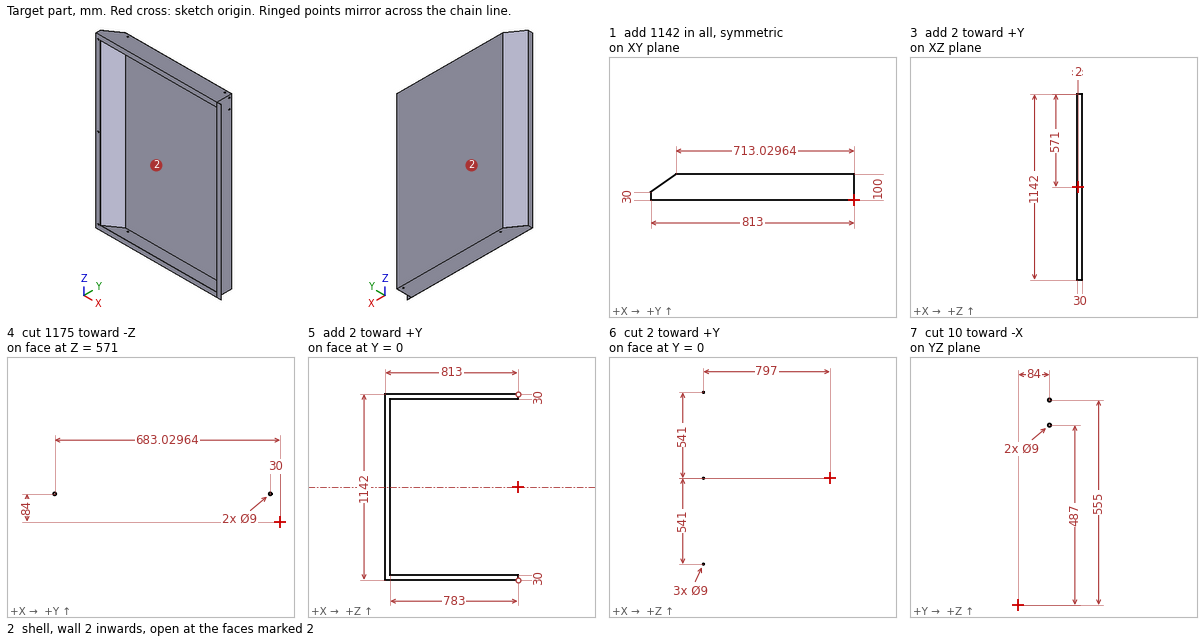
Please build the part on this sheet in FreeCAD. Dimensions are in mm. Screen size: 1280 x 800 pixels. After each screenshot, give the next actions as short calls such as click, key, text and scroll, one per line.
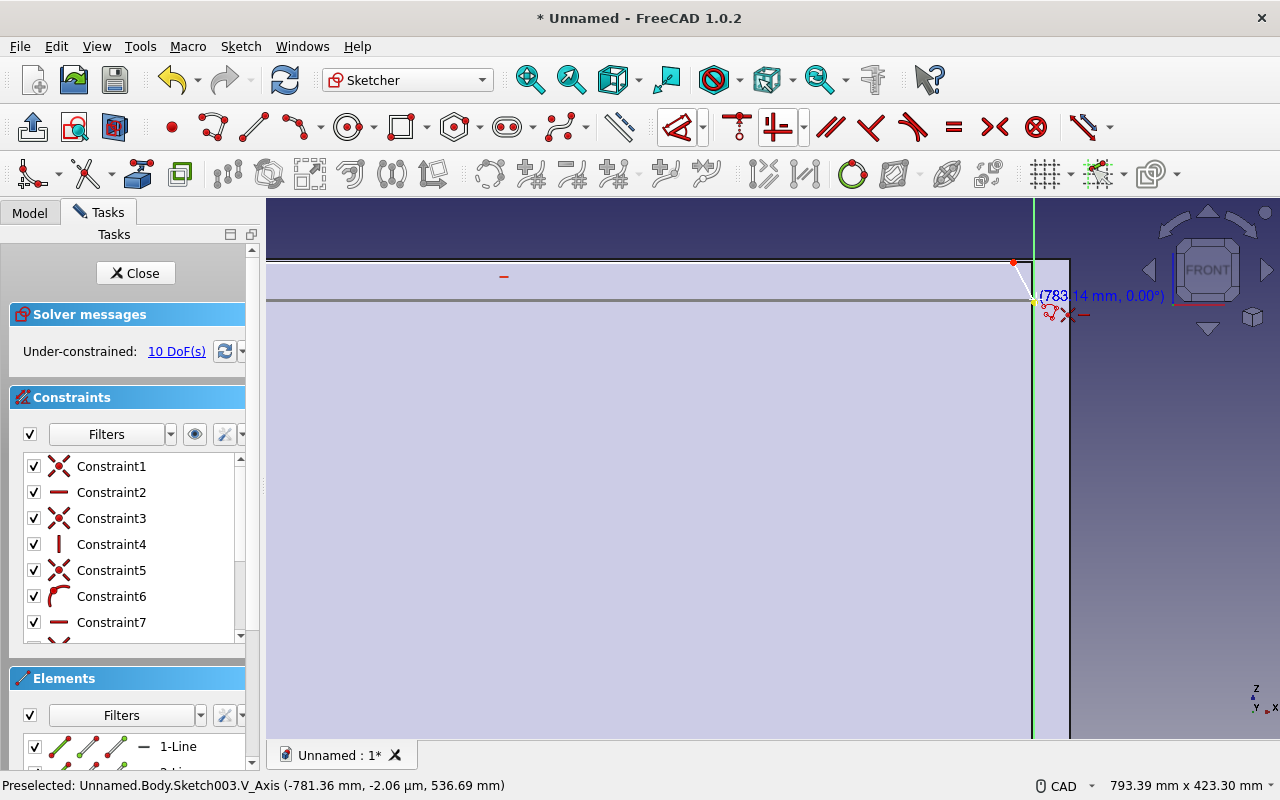
click(1035, 302)
key(Escape)
key(Escape)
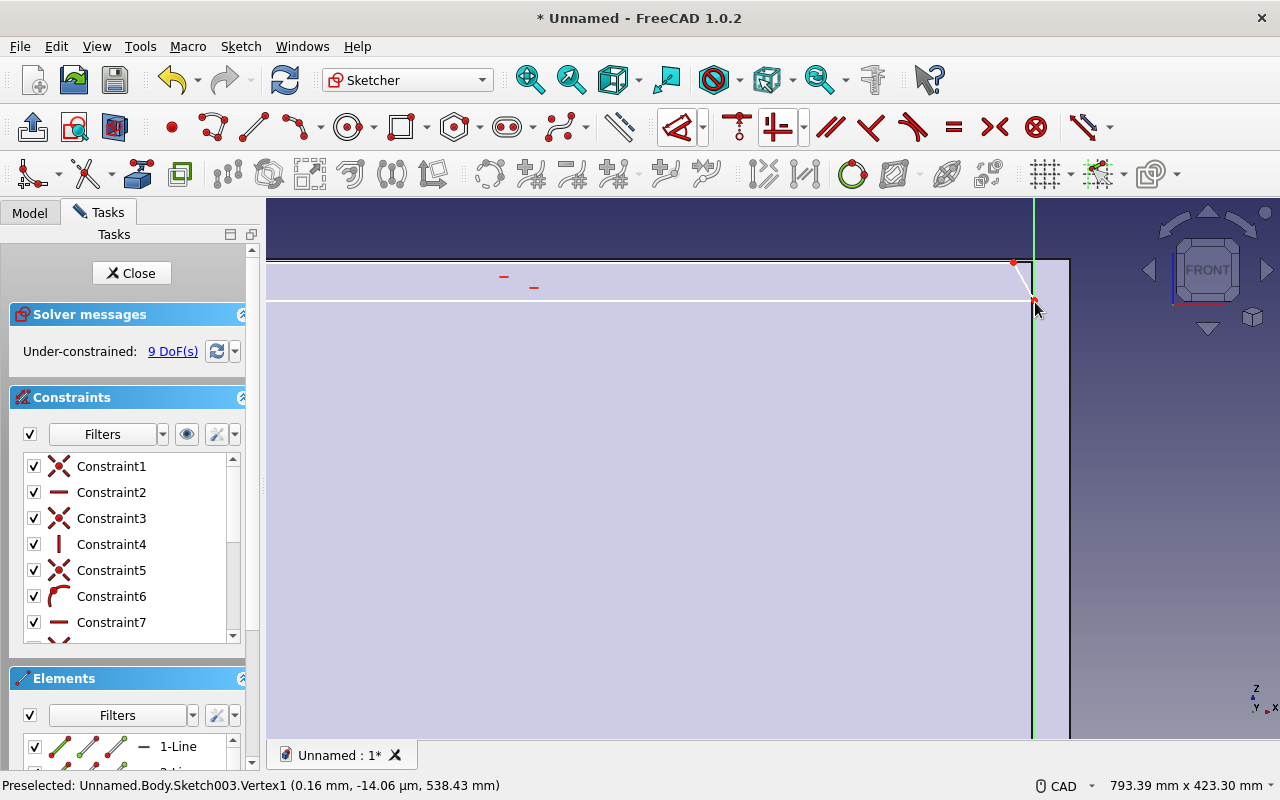
click(1020, 274)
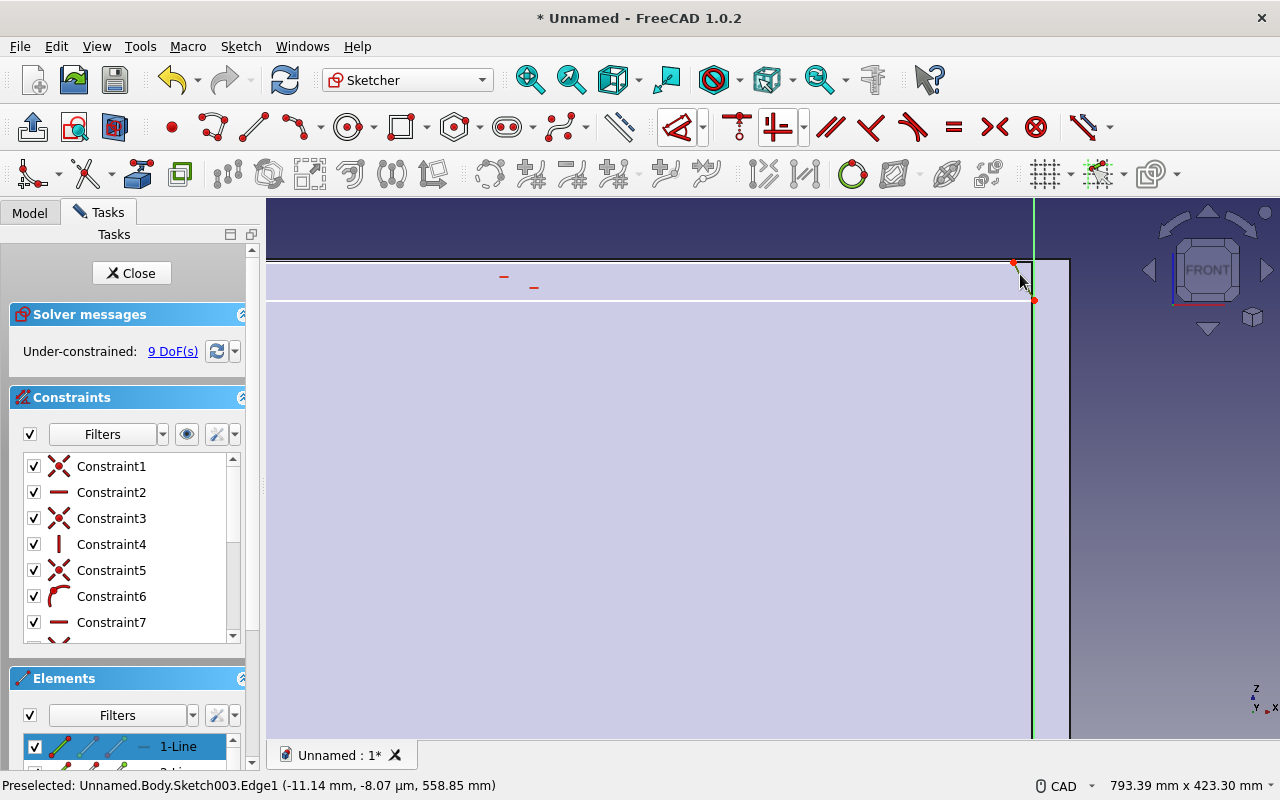
key(v)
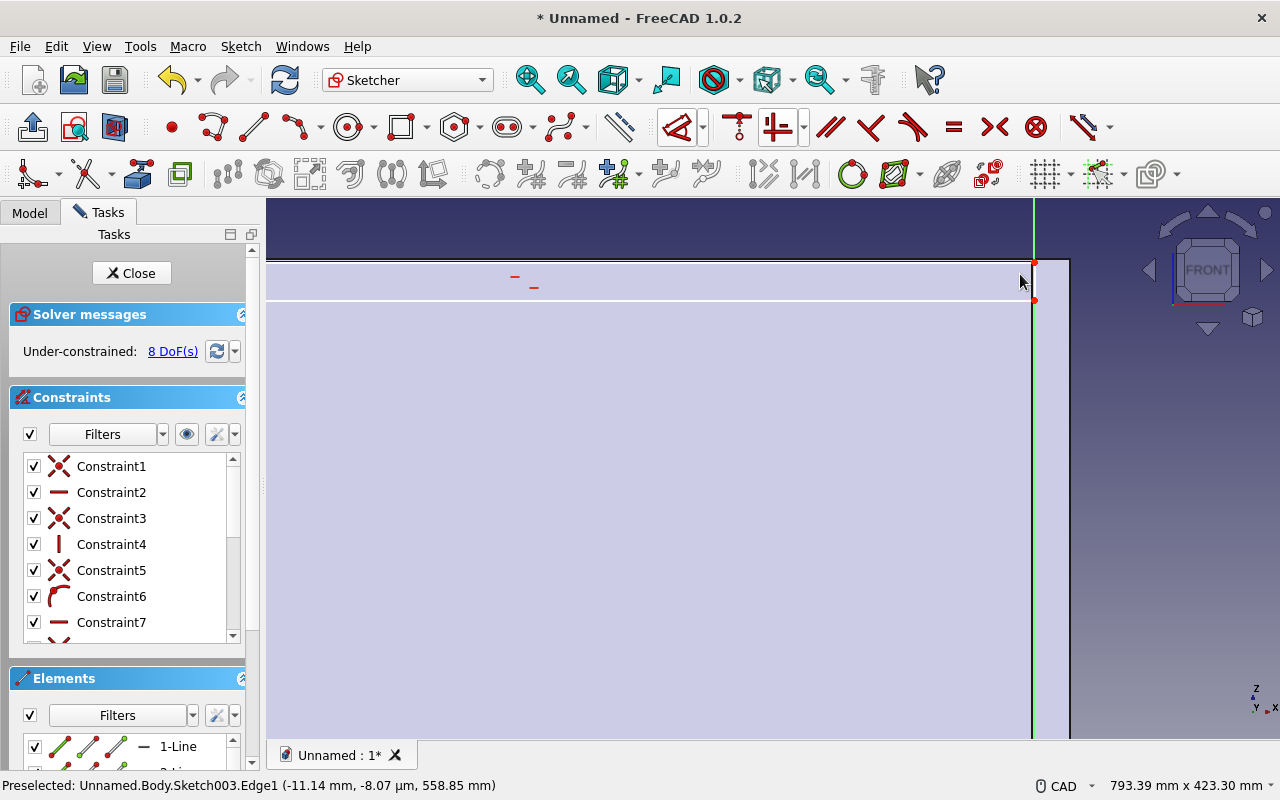
scroll(767, 298, down, 7)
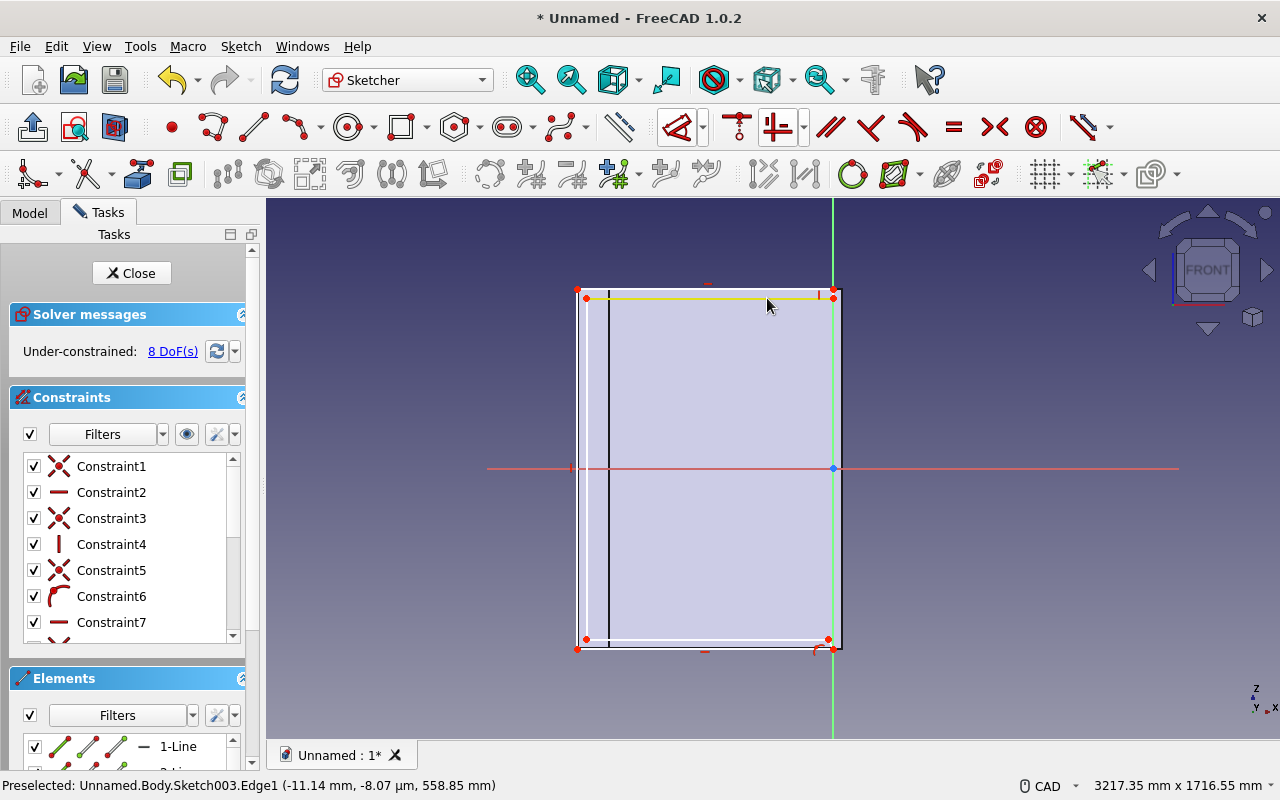
scroll(830, 642, up, 8)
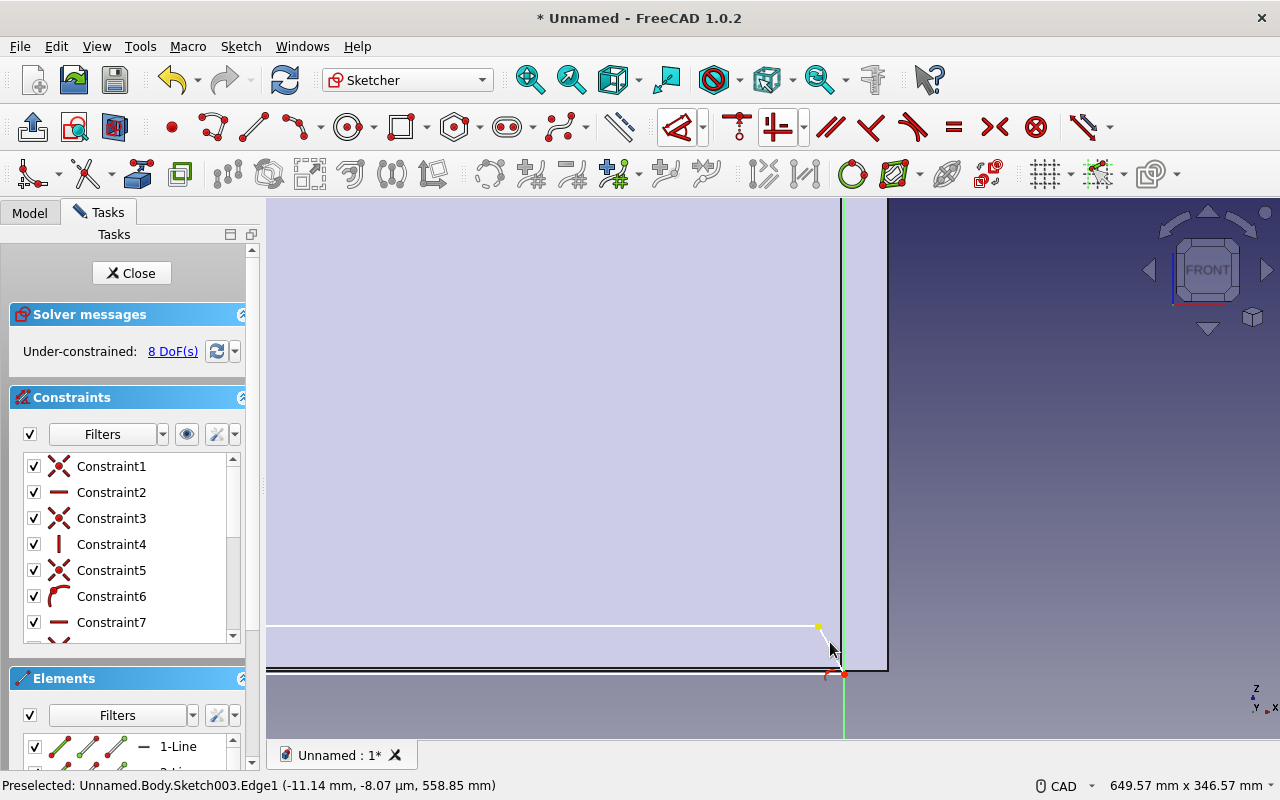
click(826, 641)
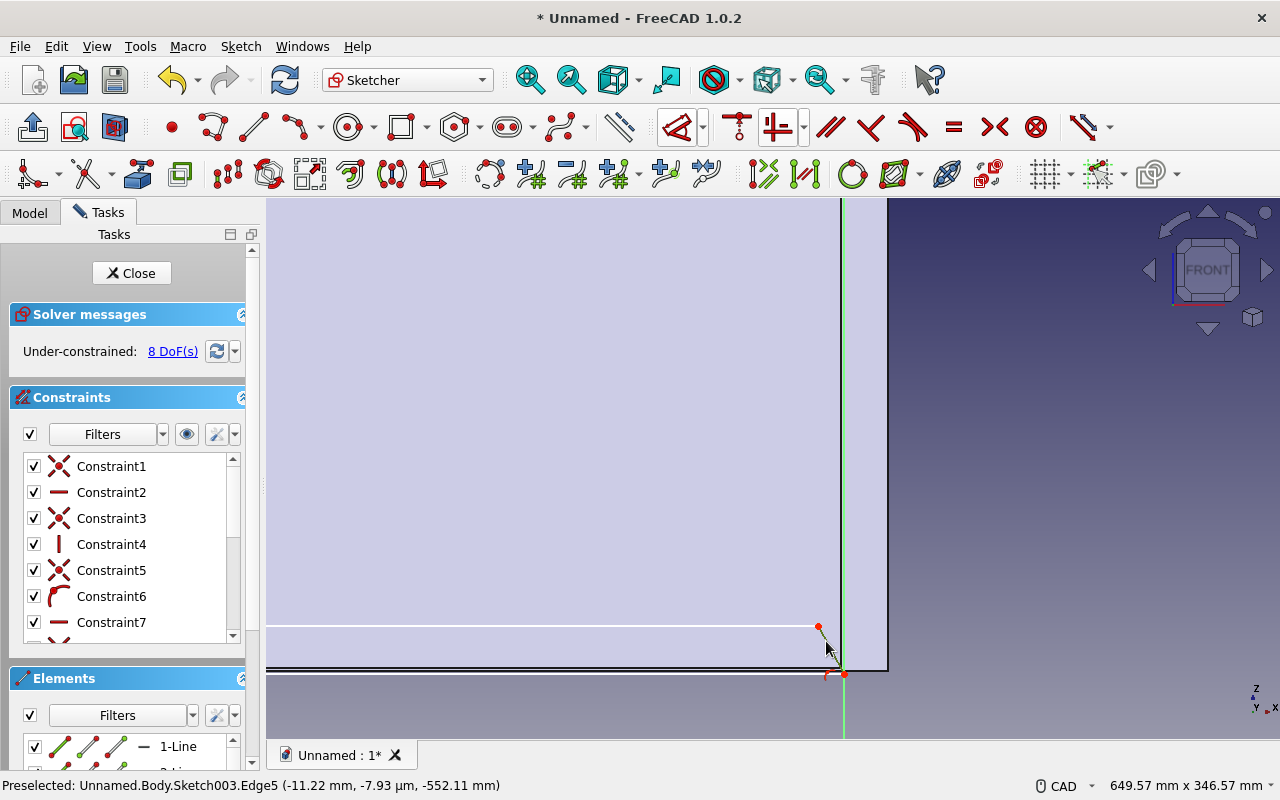
key(v)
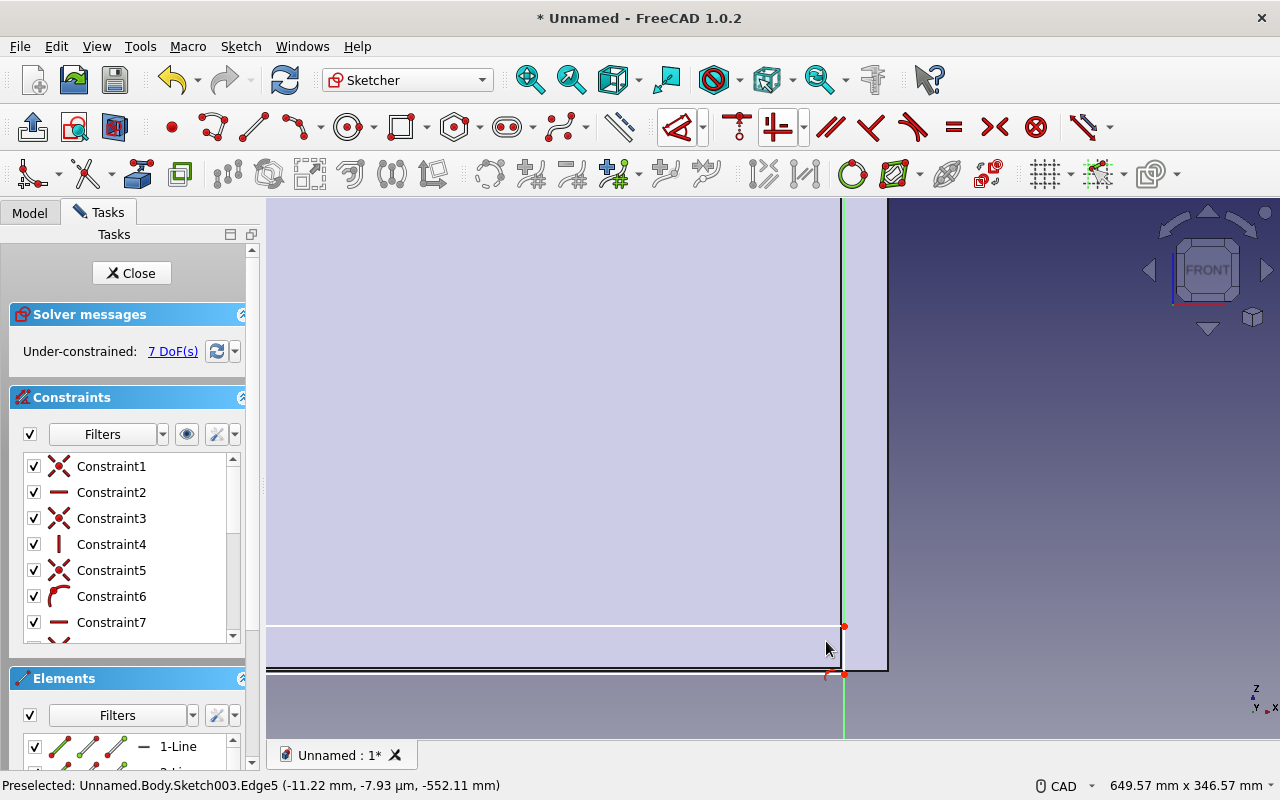
scroll(830, 643, down, 8)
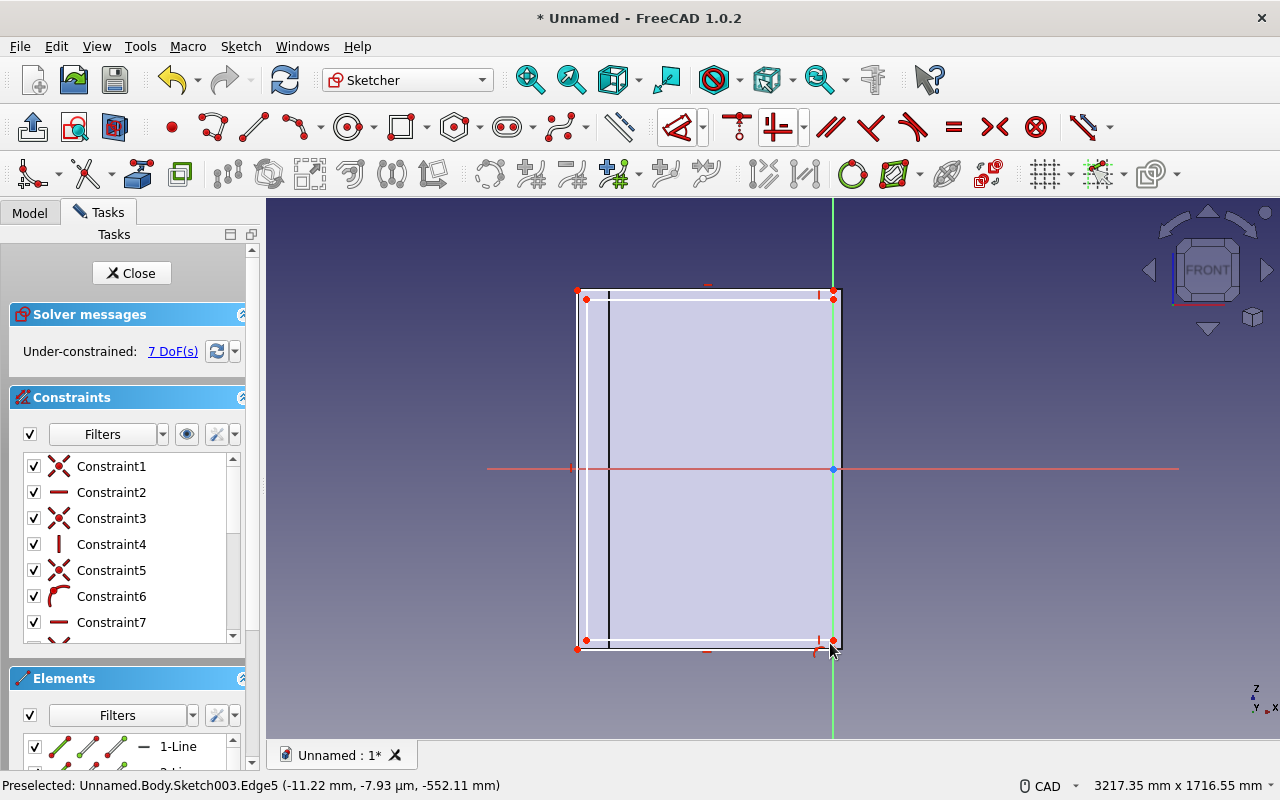
scroll(833, 290, up, 2)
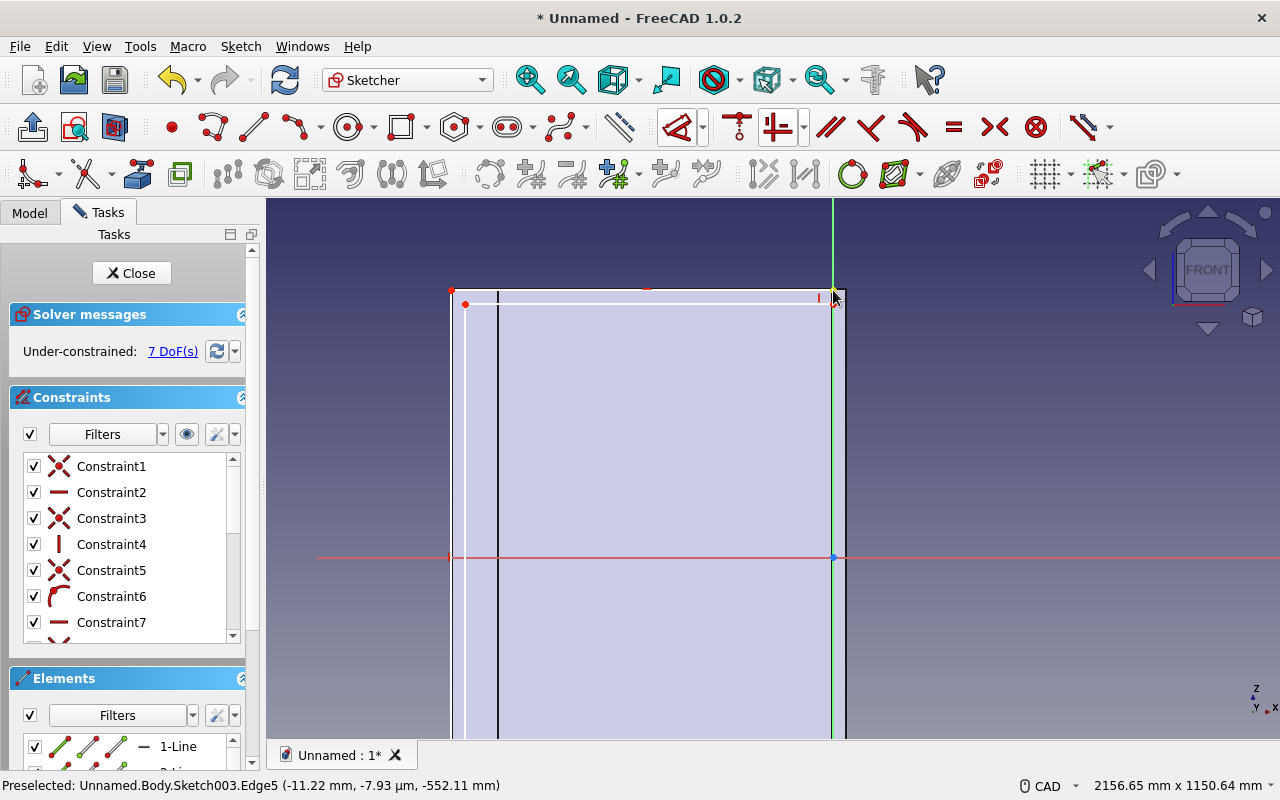
click(833, 290)